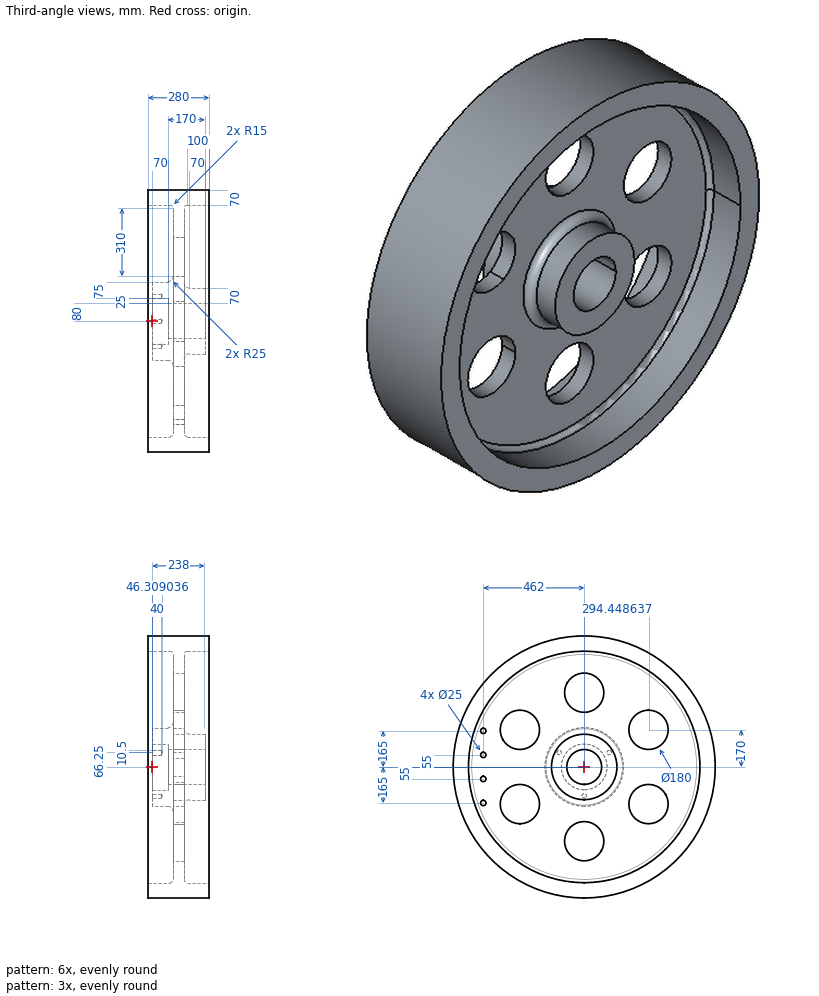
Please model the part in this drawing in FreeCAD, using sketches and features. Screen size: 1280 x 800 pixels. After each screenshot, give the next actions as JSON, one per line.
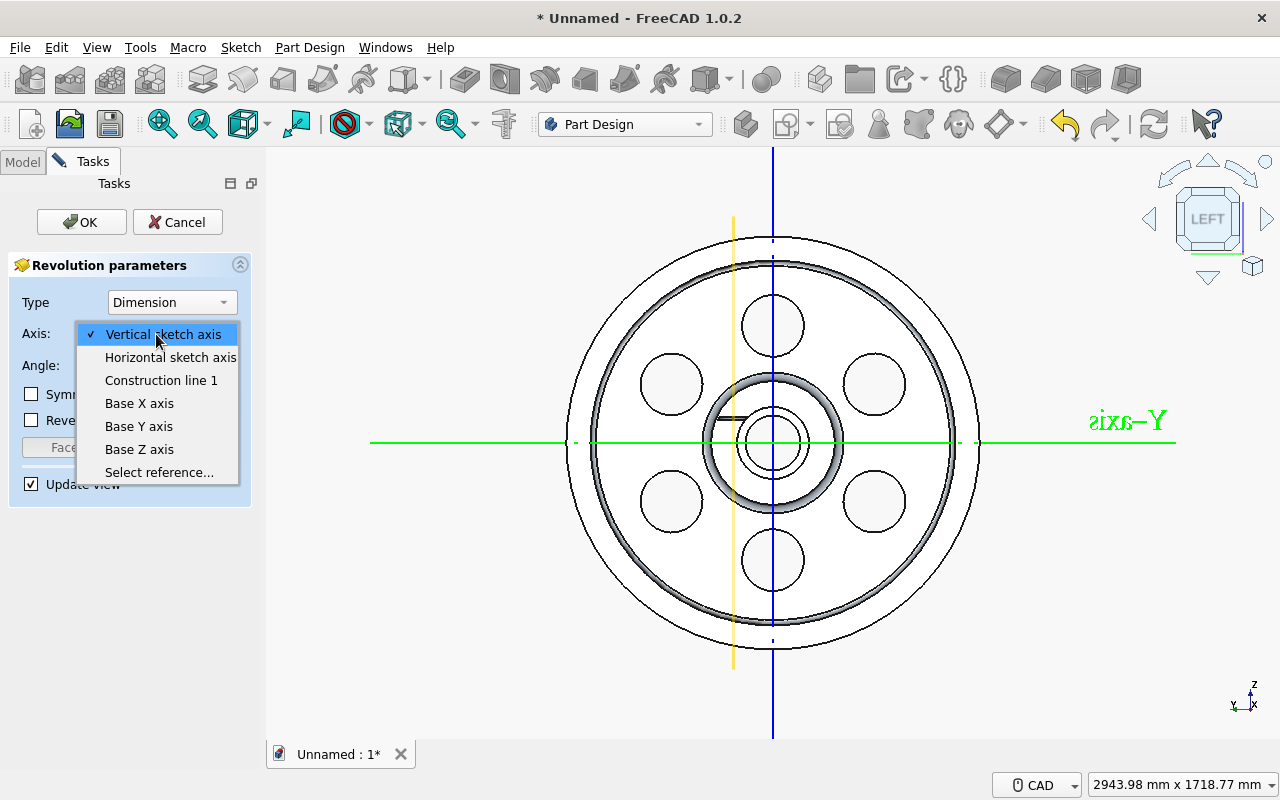
{"action": "left_click", "coordinate": [156, 380]}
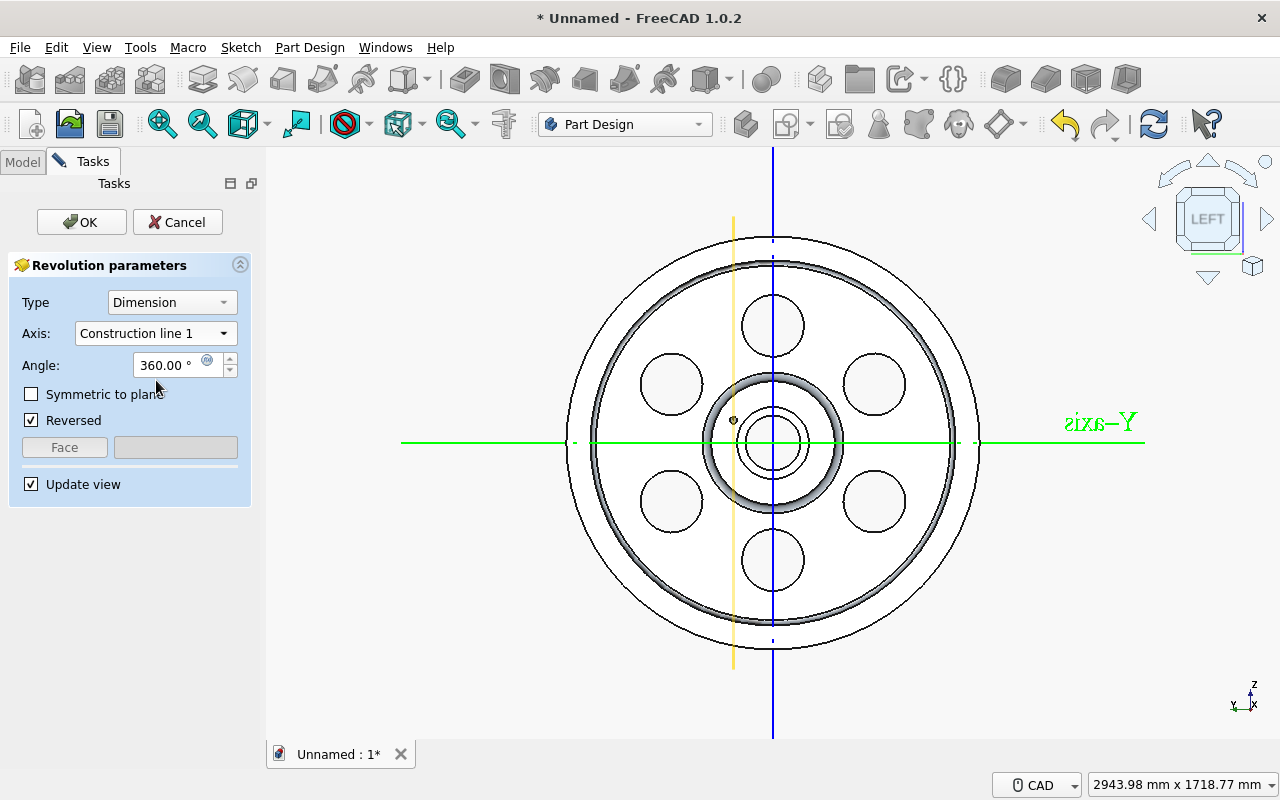
{"action": "left_click", "coordinate": [82, 222]}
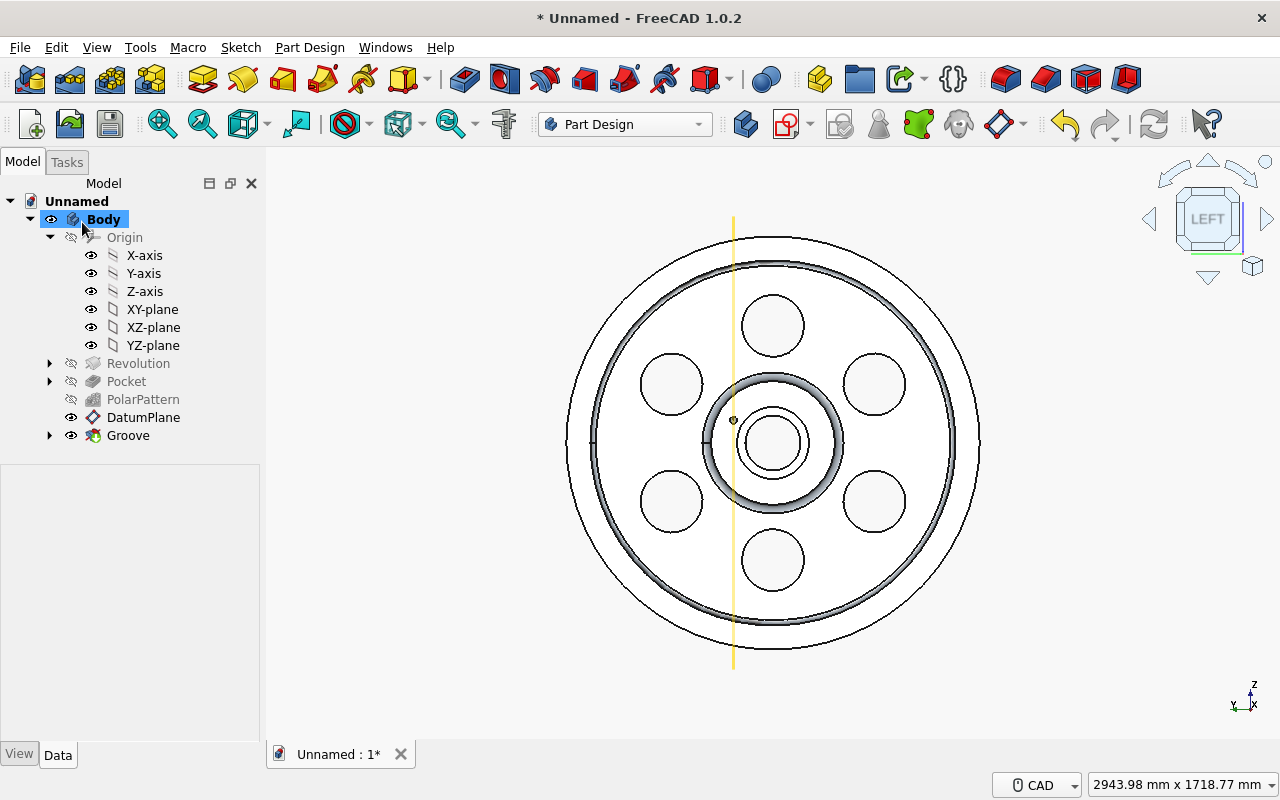
{"action": "left_click", "coordinate": [116, 417]}
{"action": "key", "text": "space"}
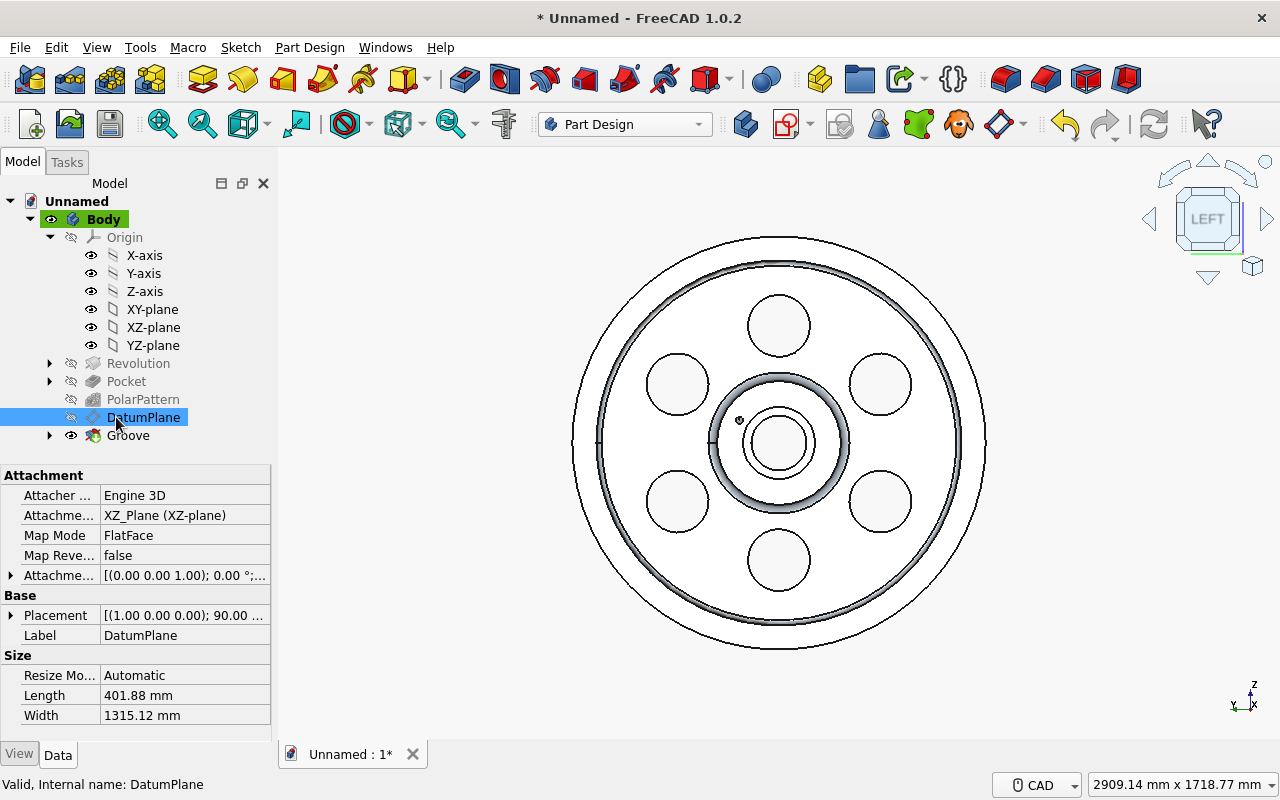
{"action": "left_click", "coordinate": [116, 435]}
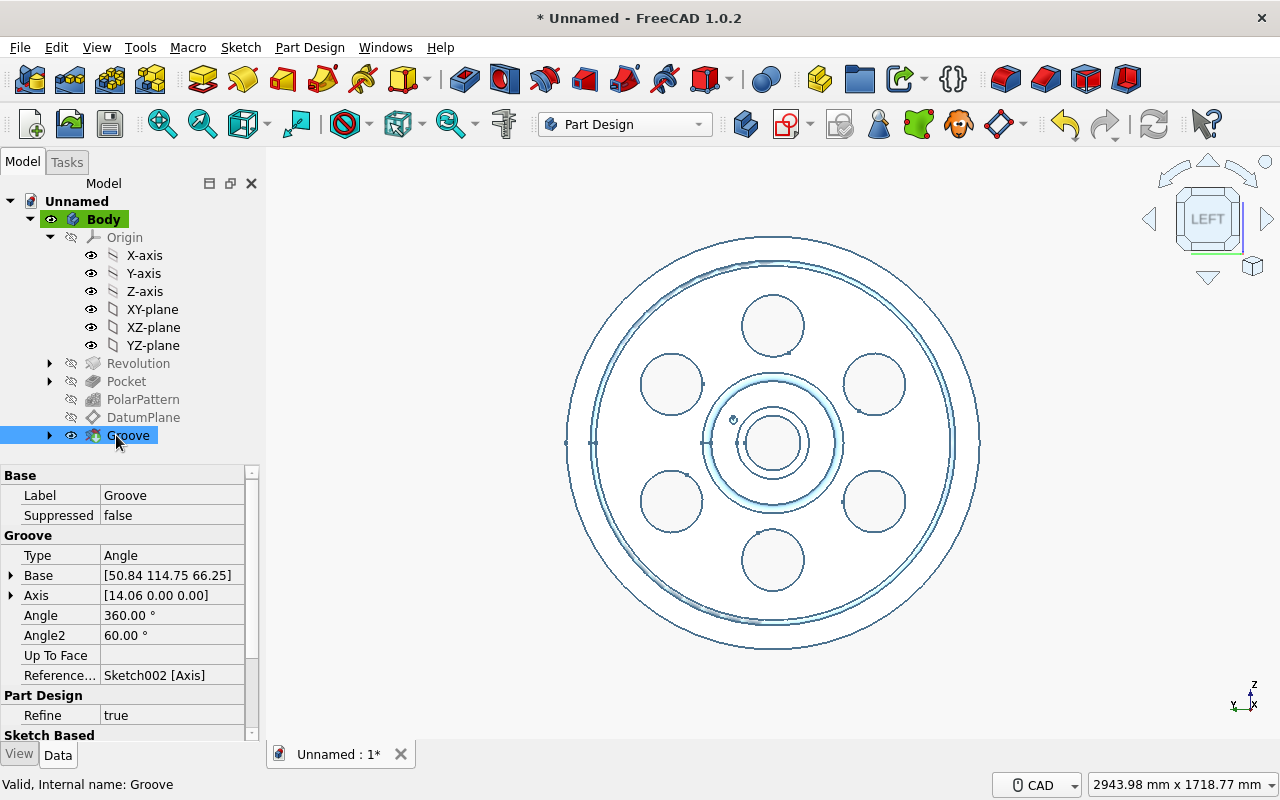
{"action": "left_click", "coordinate": [110, 80]}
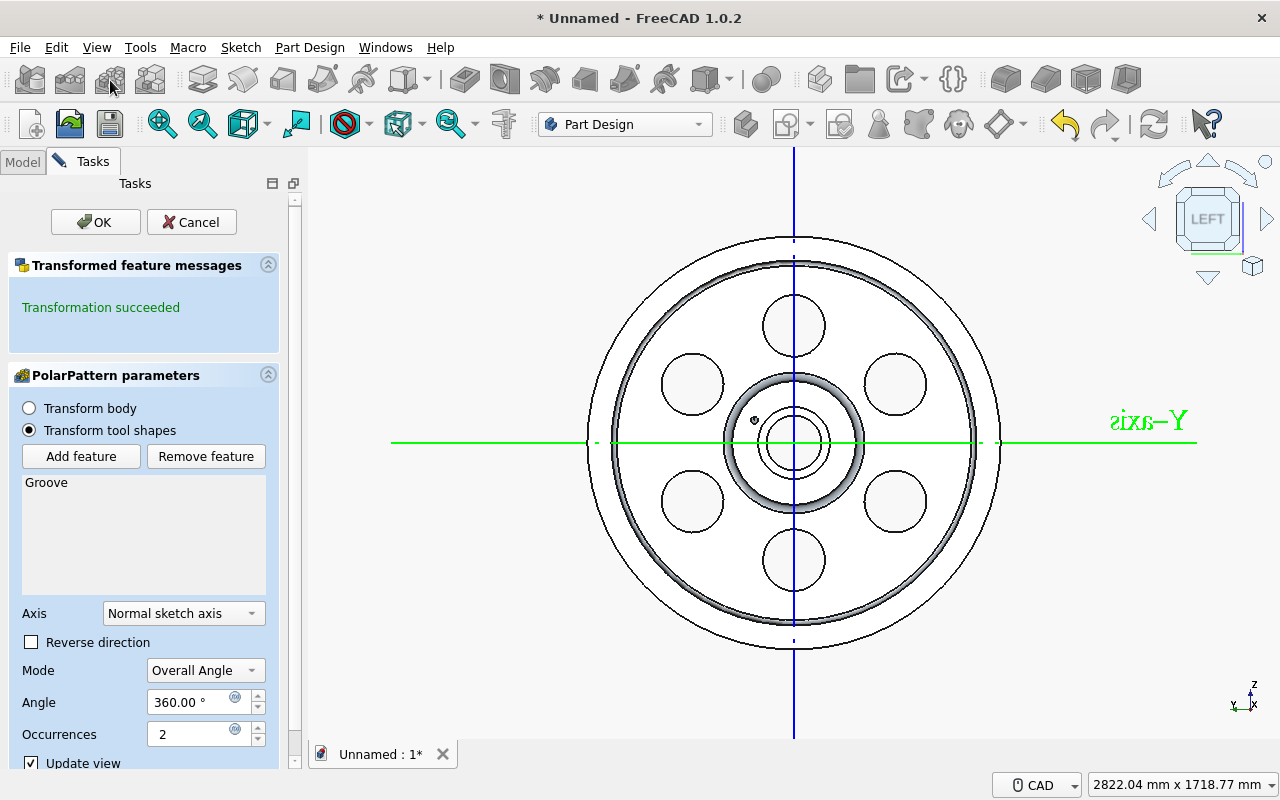
{"action": "left_click", "coordinate": [184, 614]}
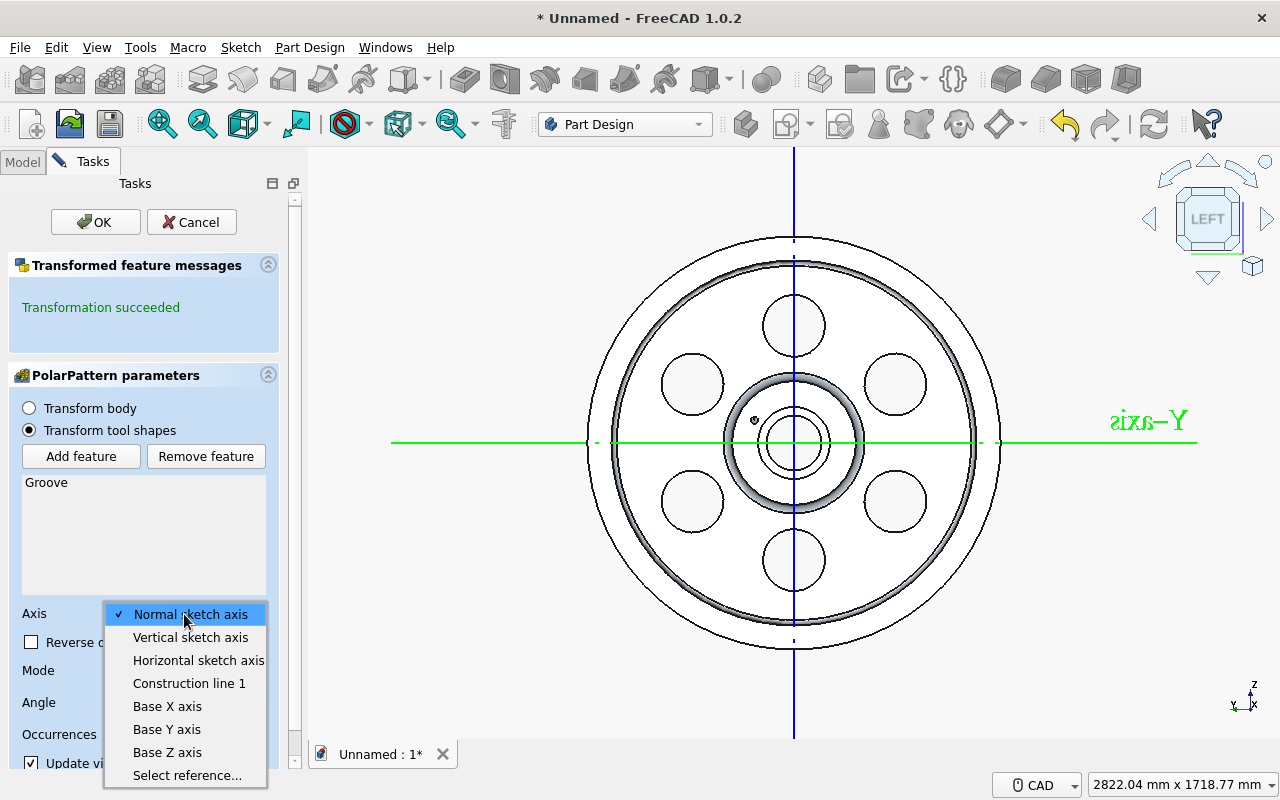
{"action": "left_click", "coordinate": [184, 706]}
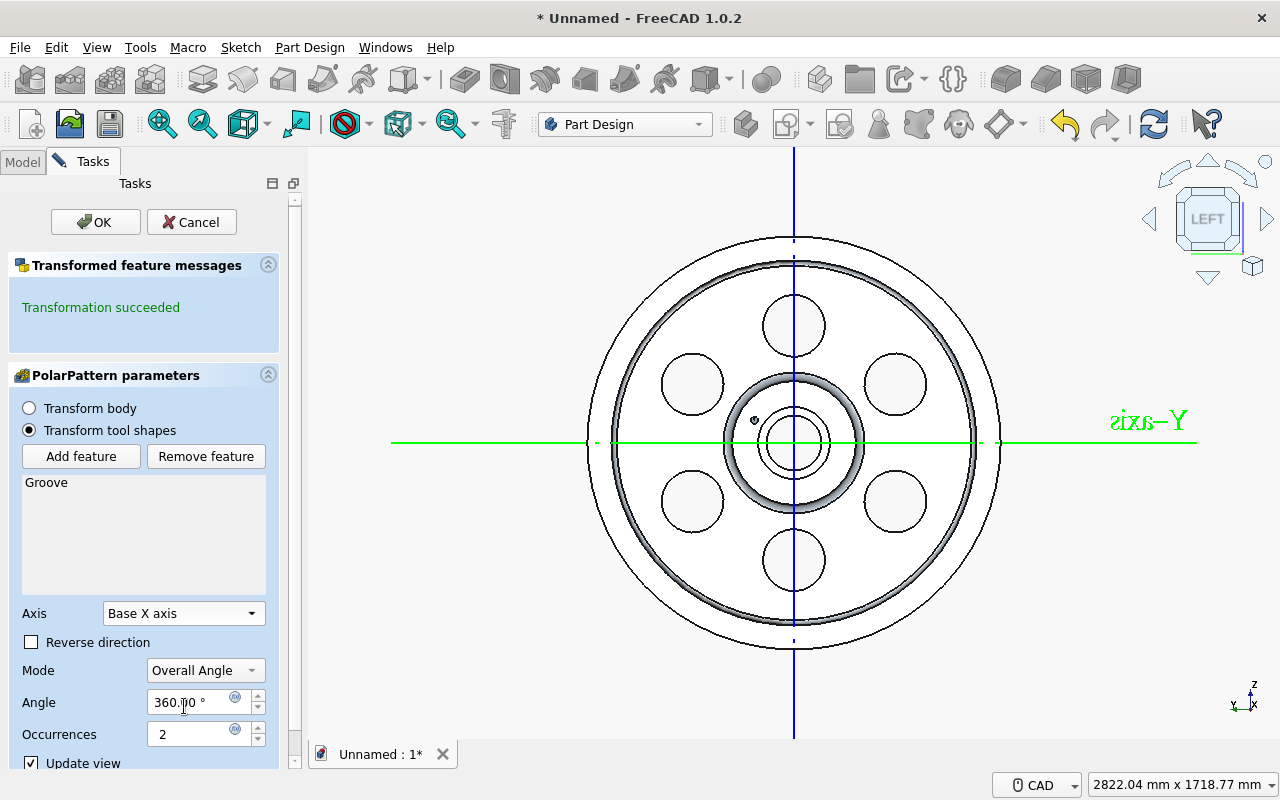
{"action": "triple_click", "coordinate": [198, 734]}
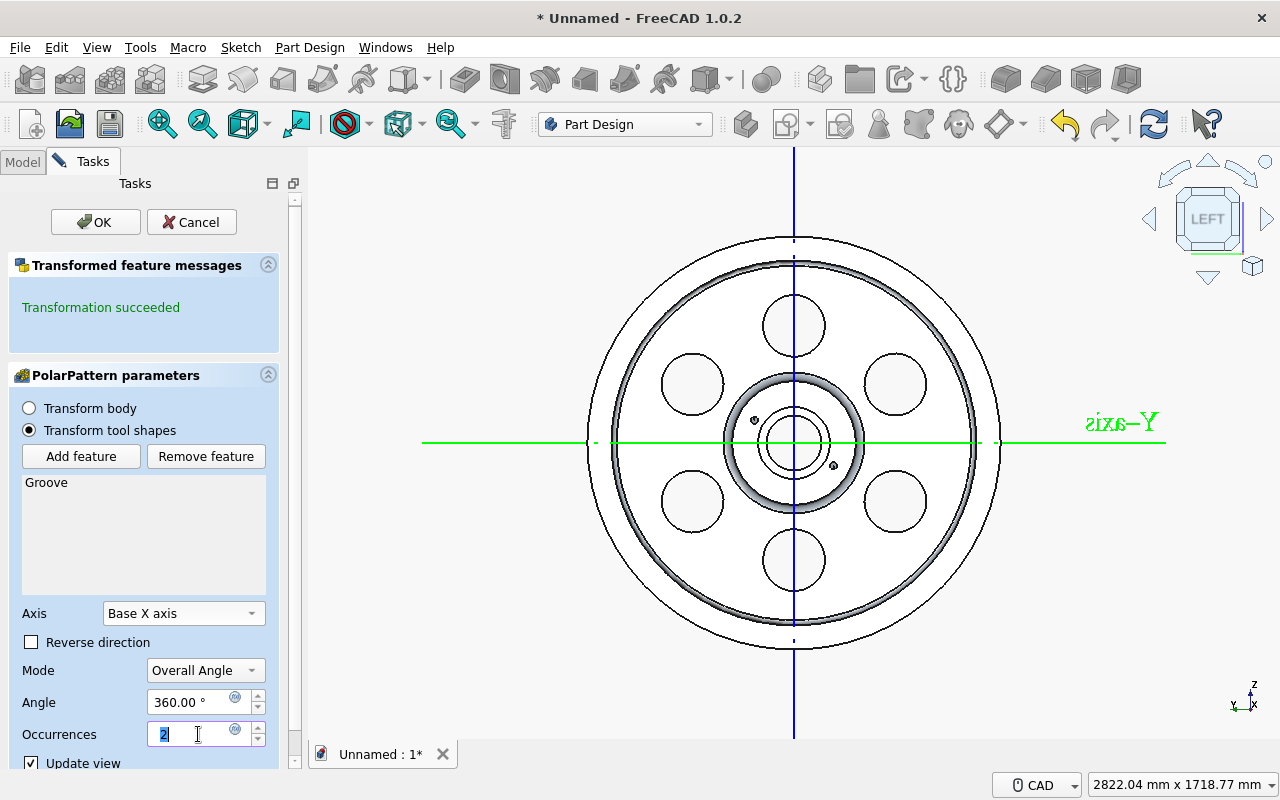
{"action": "type", "text": "3"}
{"action": "key", "text": "Tab"}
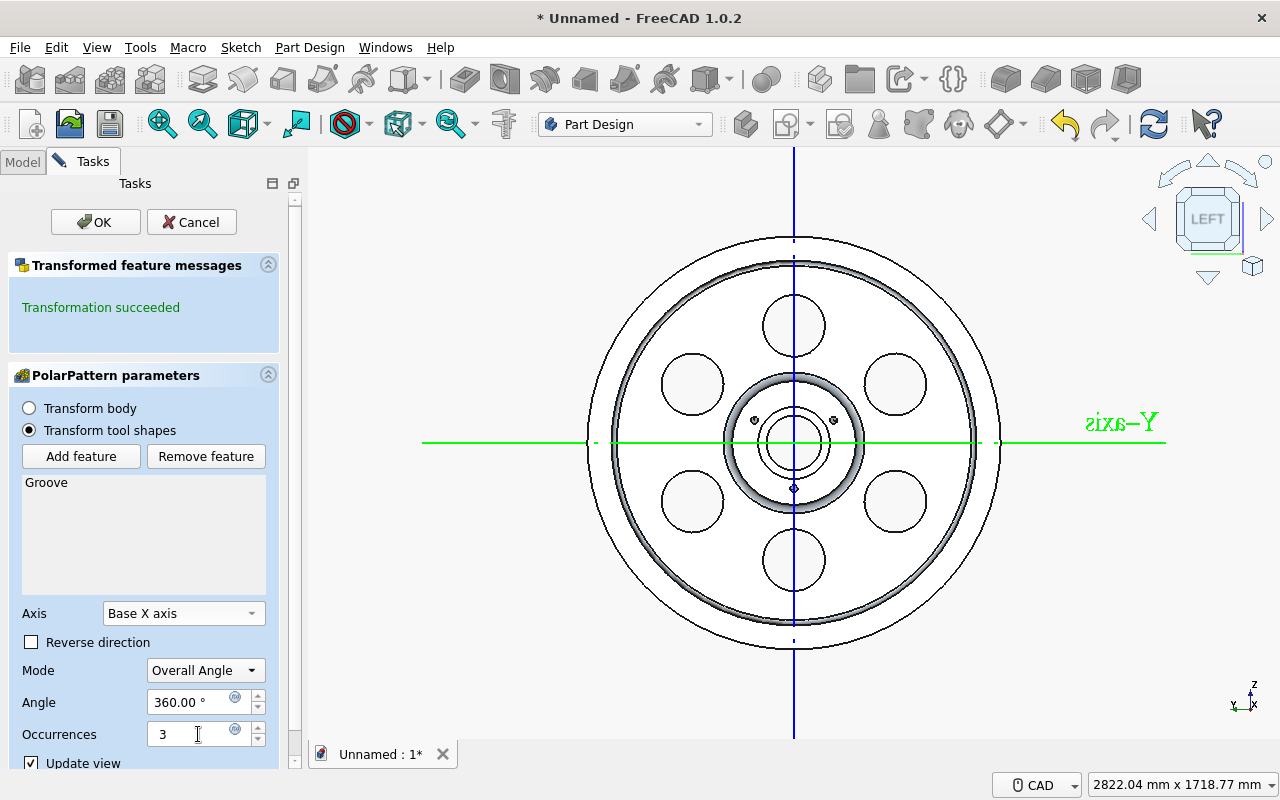
{"action": "left_click", "coordinate": [96, 222]}